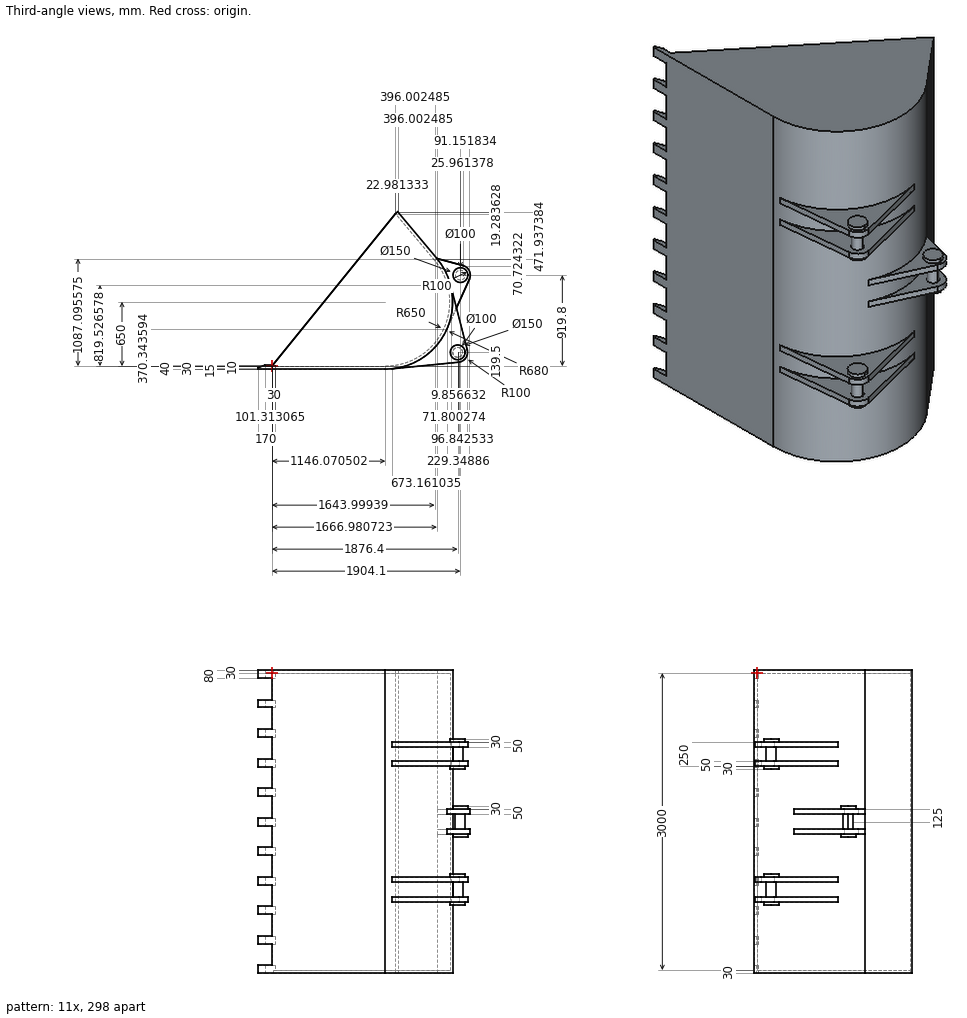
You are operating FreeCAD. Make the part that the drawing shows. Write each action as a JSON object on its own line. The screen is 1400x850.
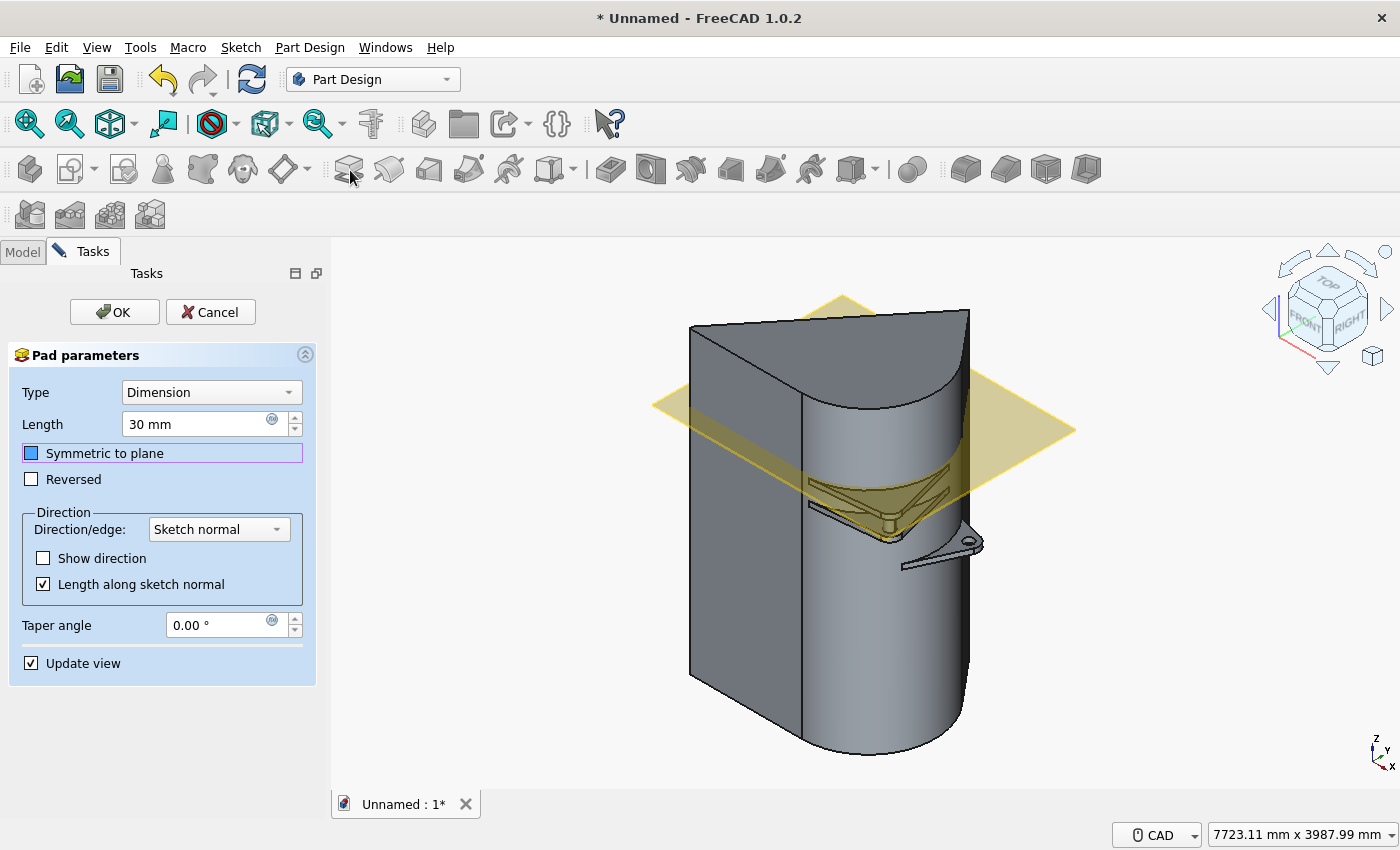
{"action": "left_click", "coordinate": [30, 479]}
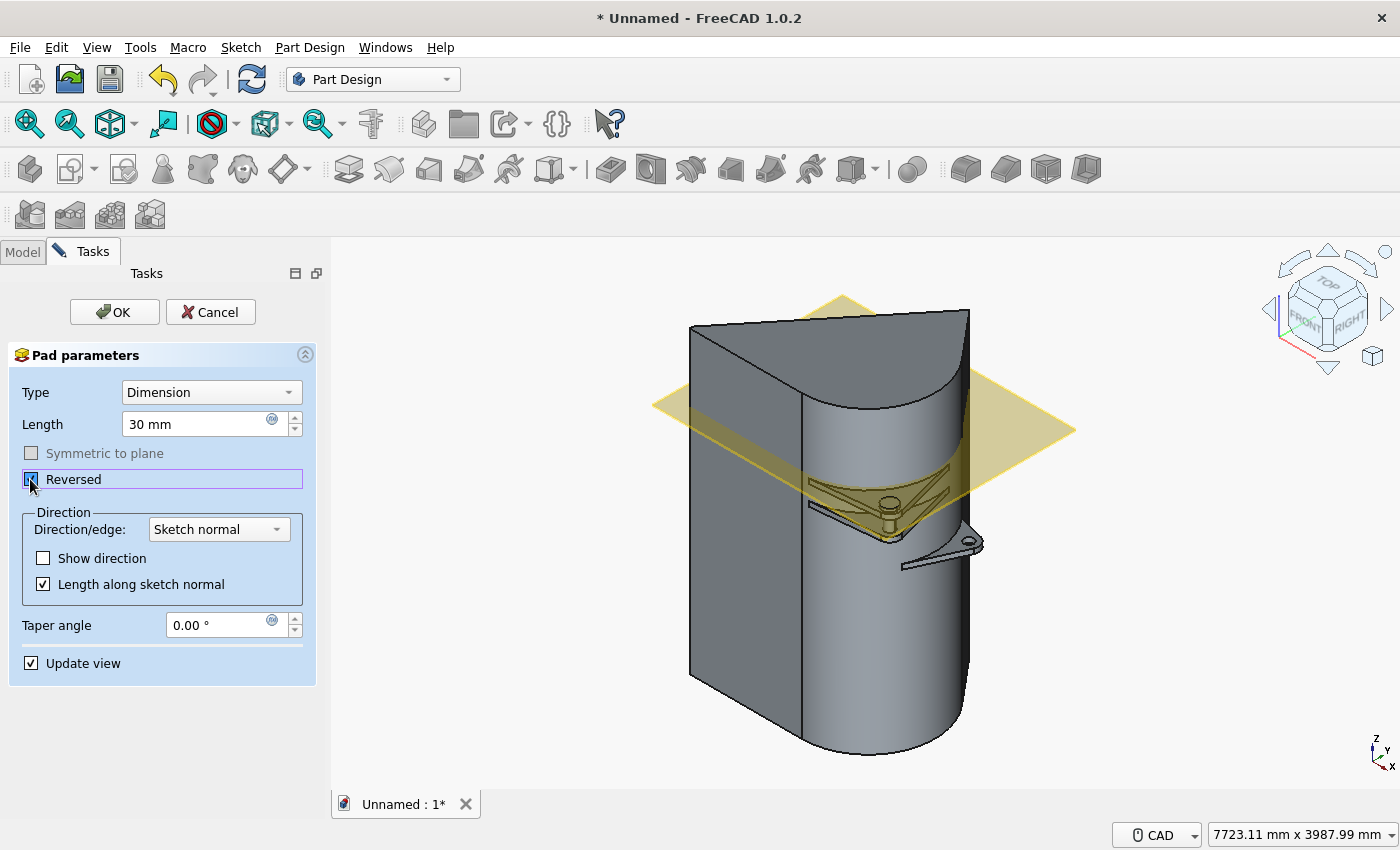
{"action": "left_click", "coordinate": [115, 312]}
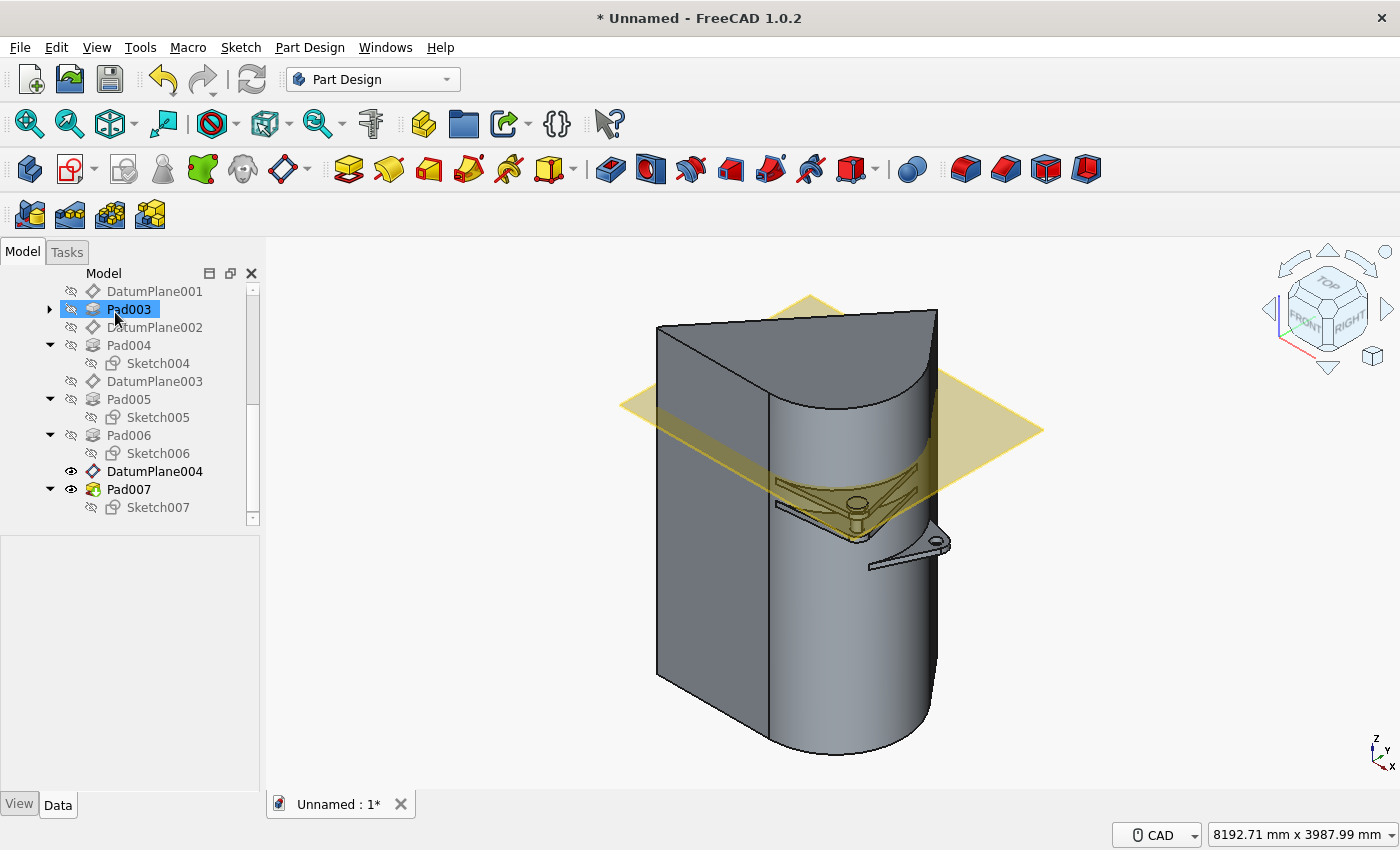
{"action": "left_click", "coordinate": [116, 471]}
{"action": "key", "text": "space"}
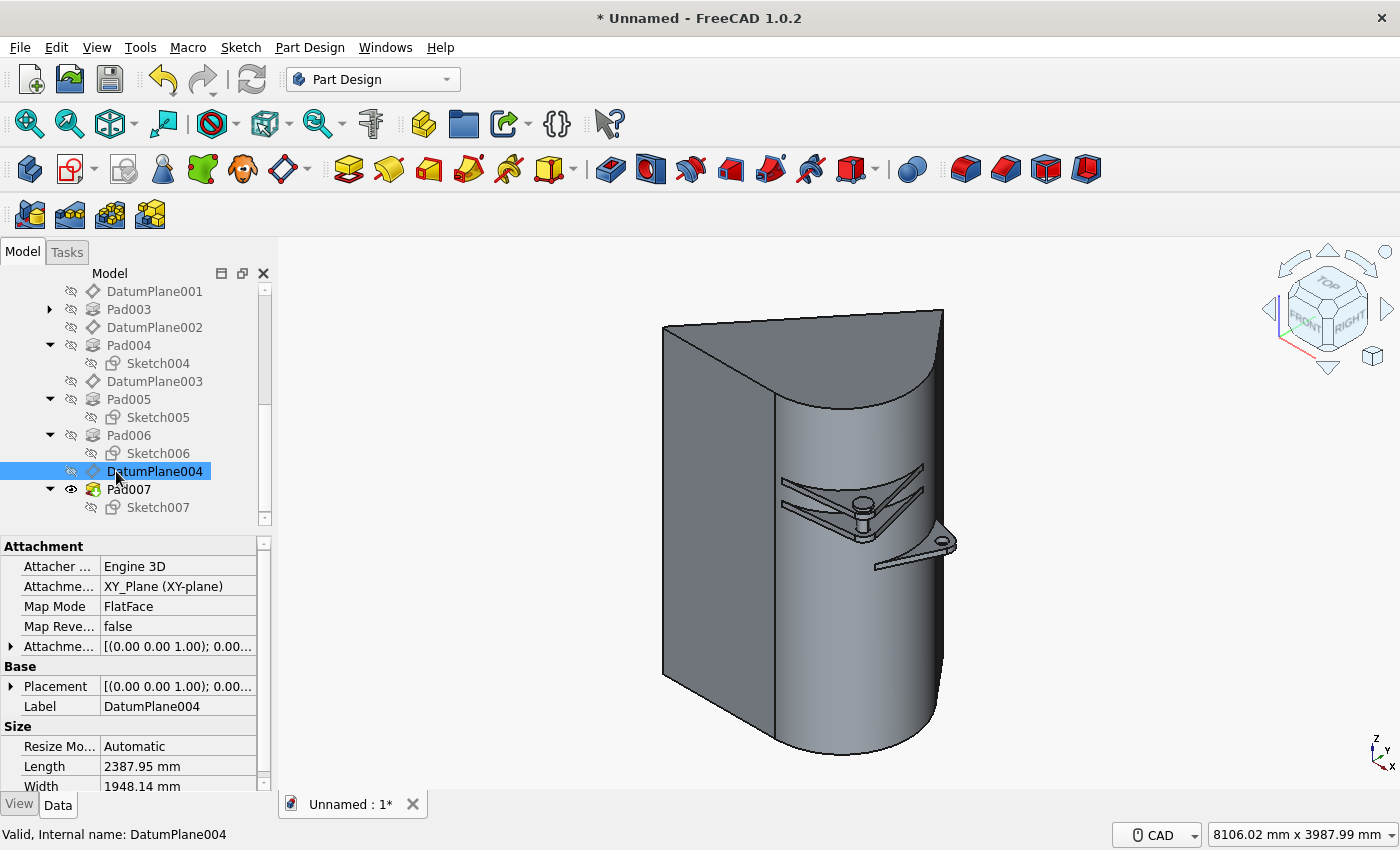
{"action": "key", "text": "5"}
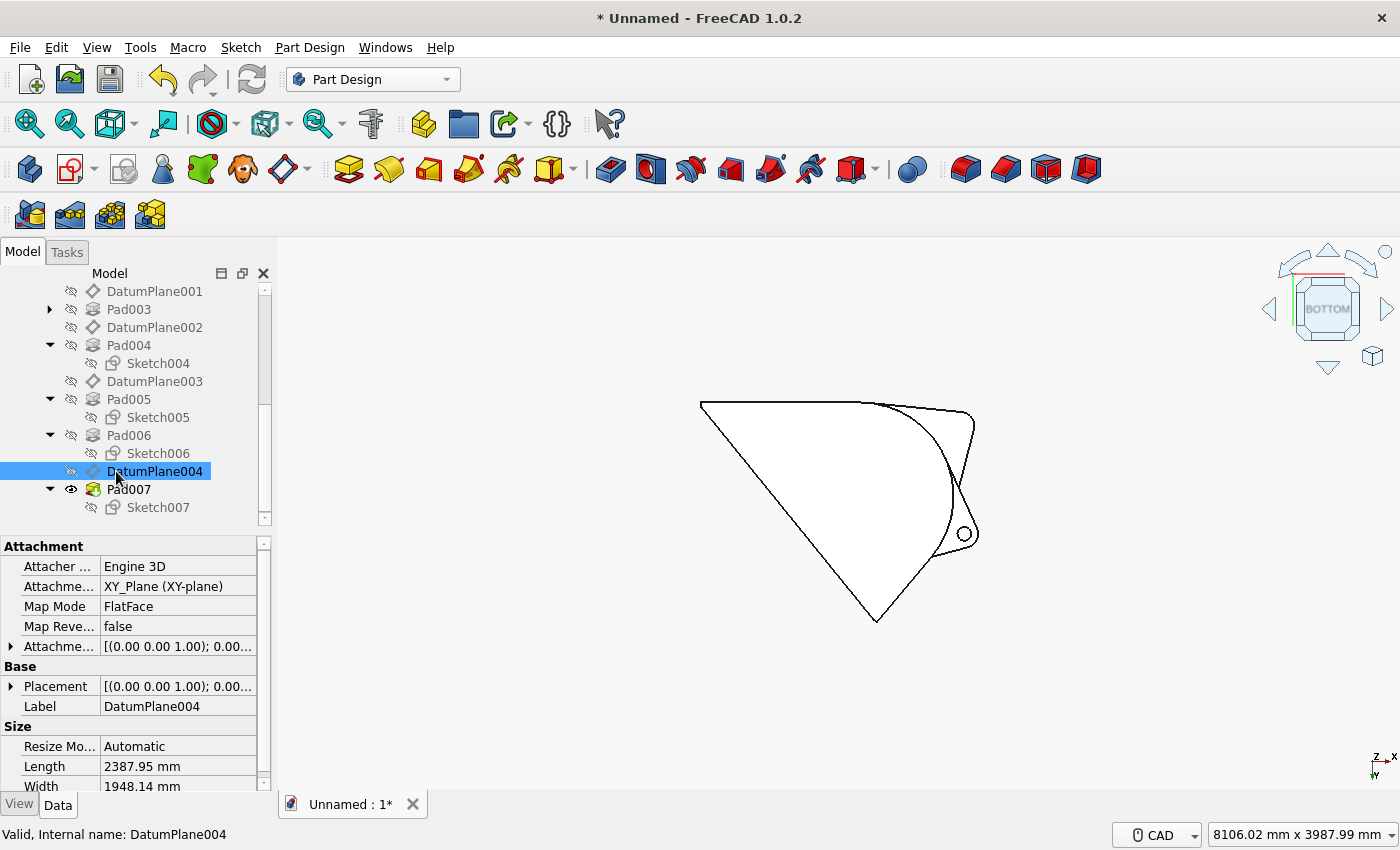
{"action": "key", "text": "v f"}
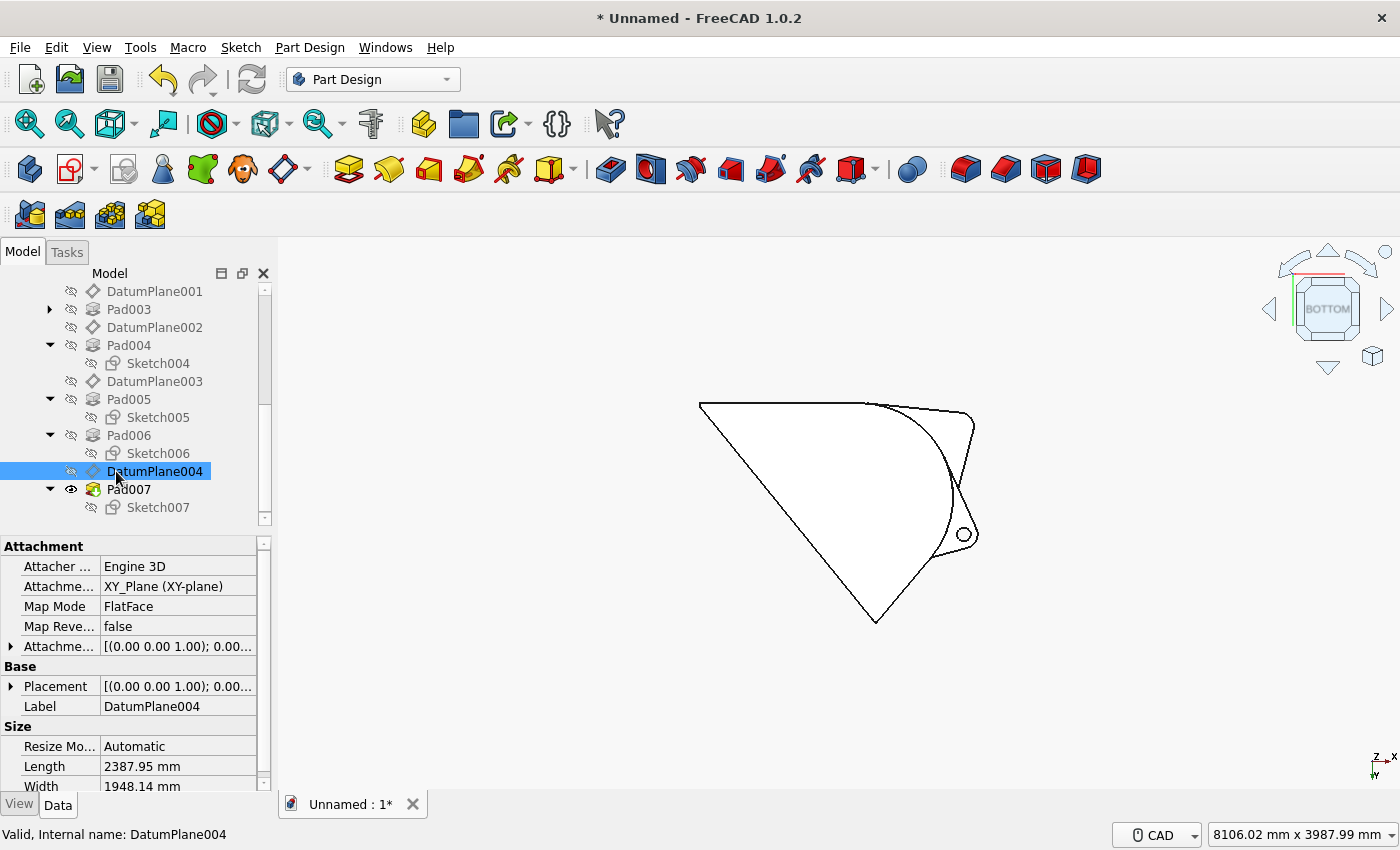
{"action": "left_click", "coordinate": [951, 428]}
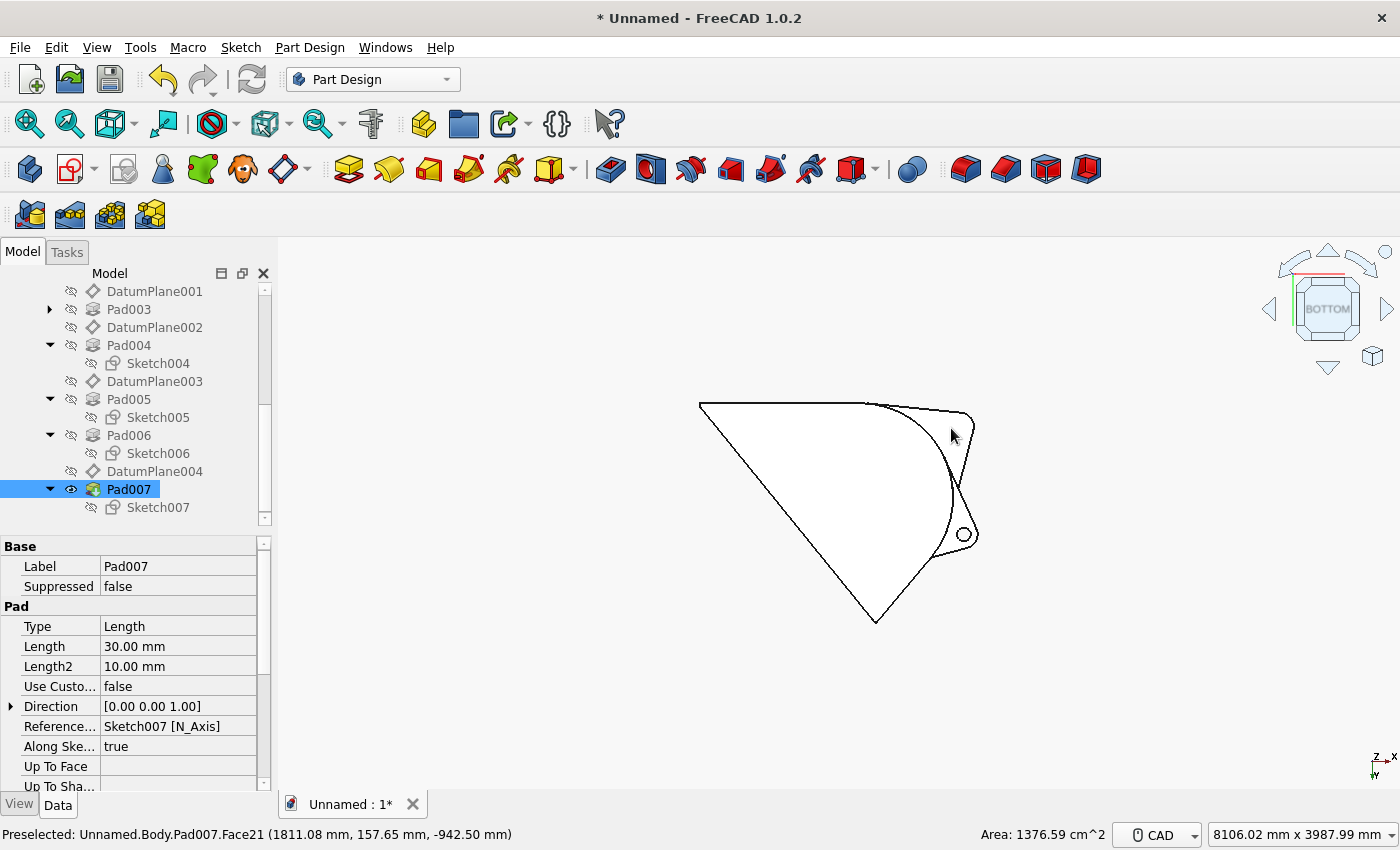
{"action": "left_click", "coordinate": [70, 170]}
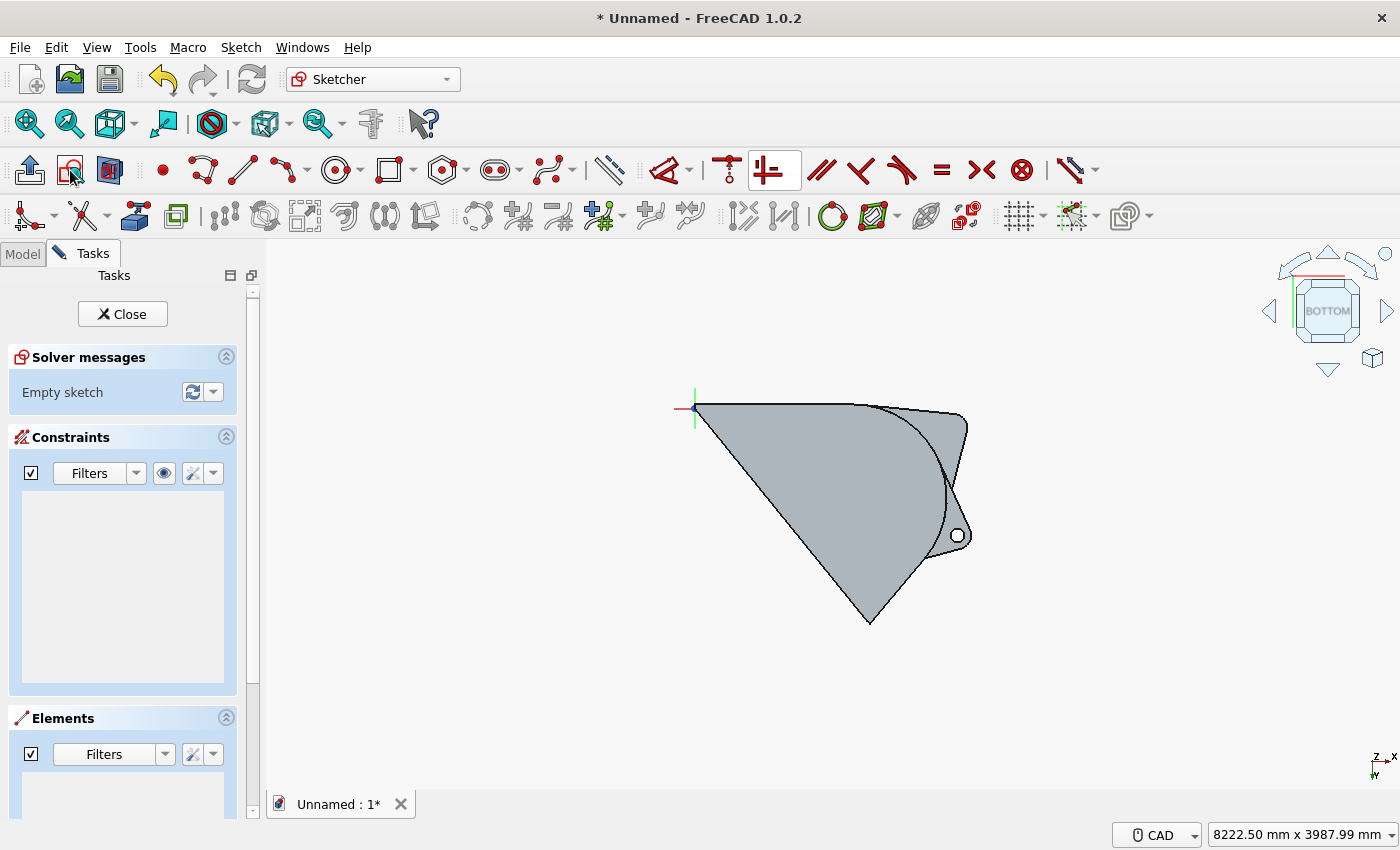
{"action": "left_click", "coordinate": [110, 170]}